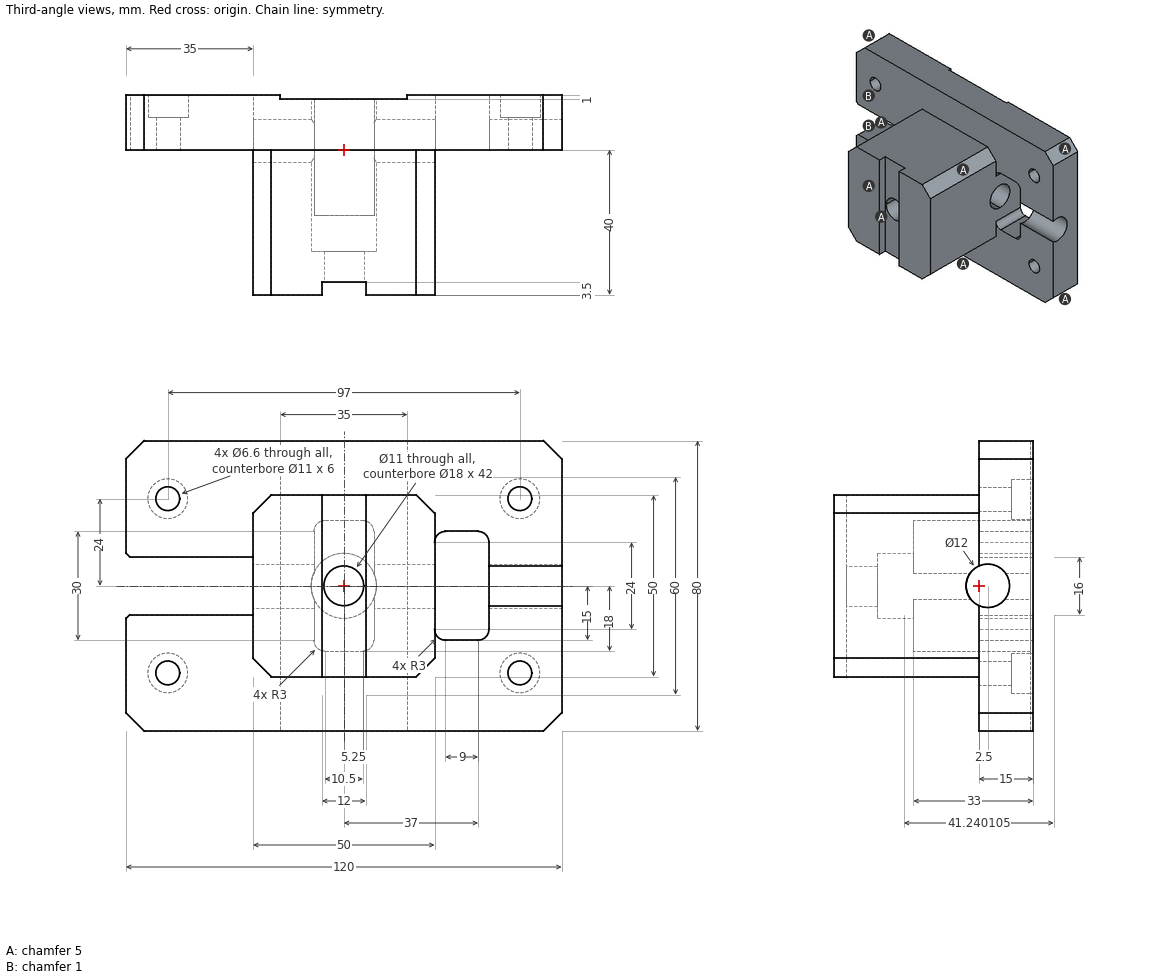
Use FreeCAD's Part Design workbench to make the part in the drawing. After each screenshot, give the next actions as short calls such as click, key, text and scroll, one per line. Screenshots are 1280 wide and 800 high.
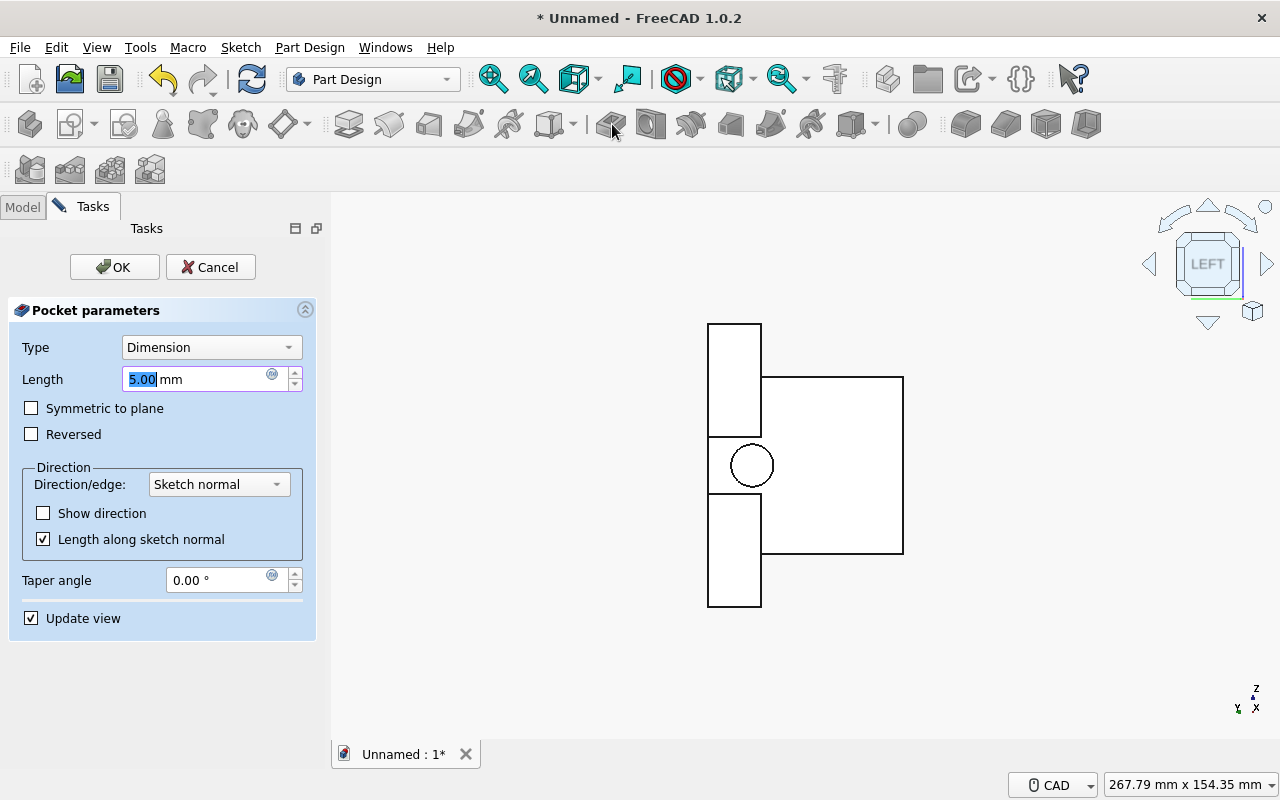
click(212, 348)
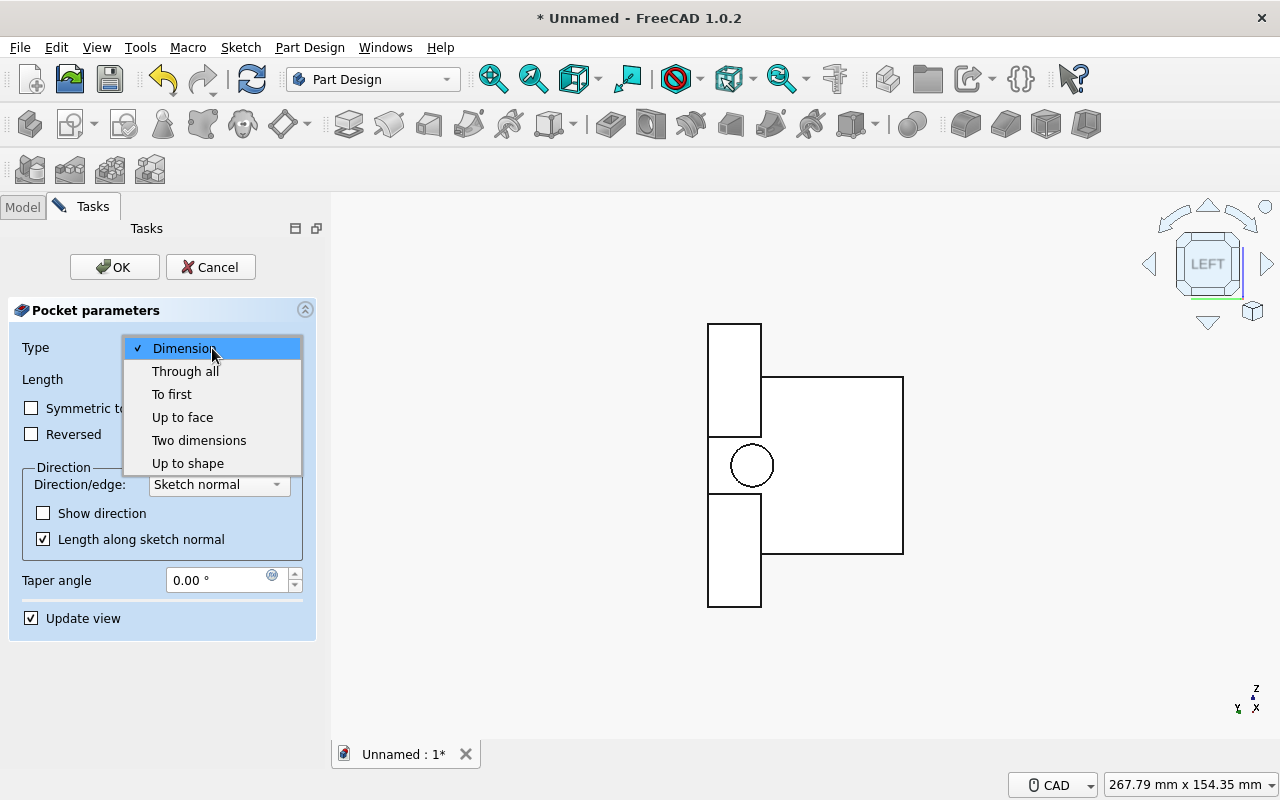
click(212, 372)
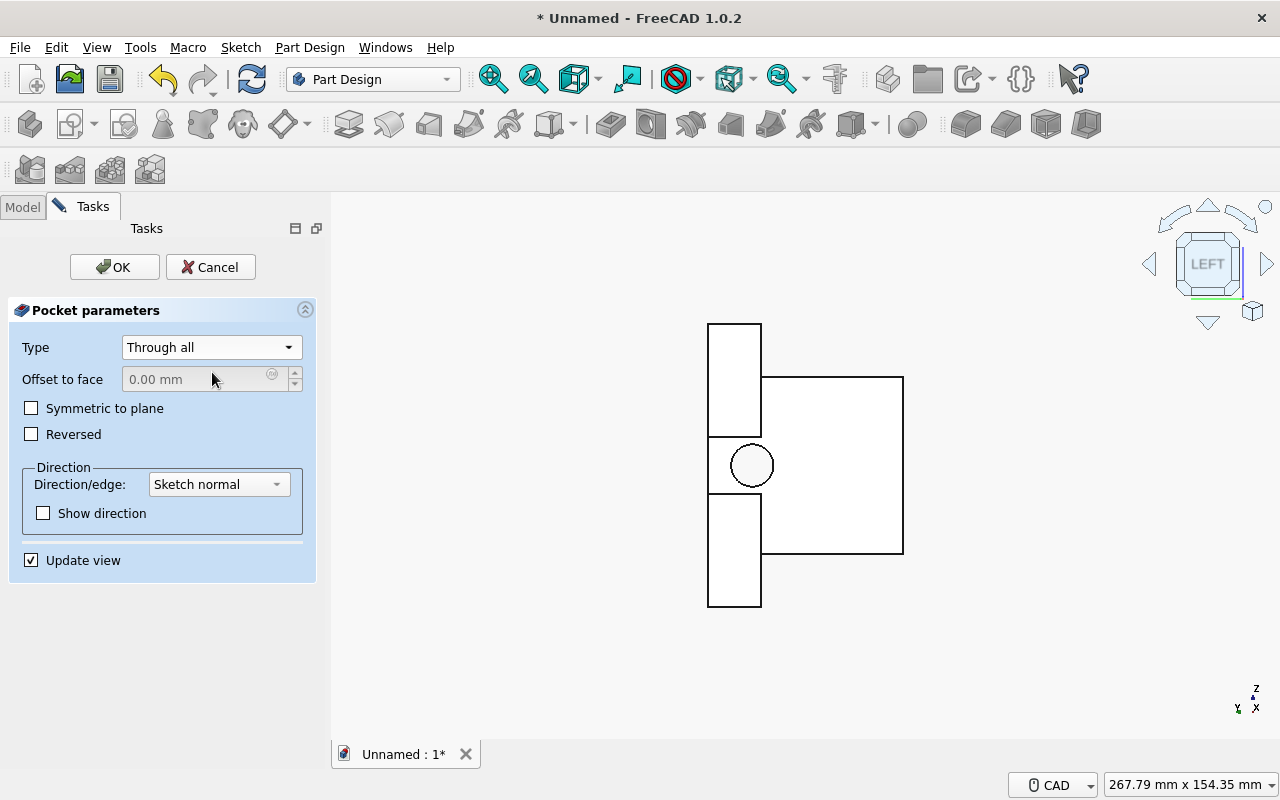
click(115, 267)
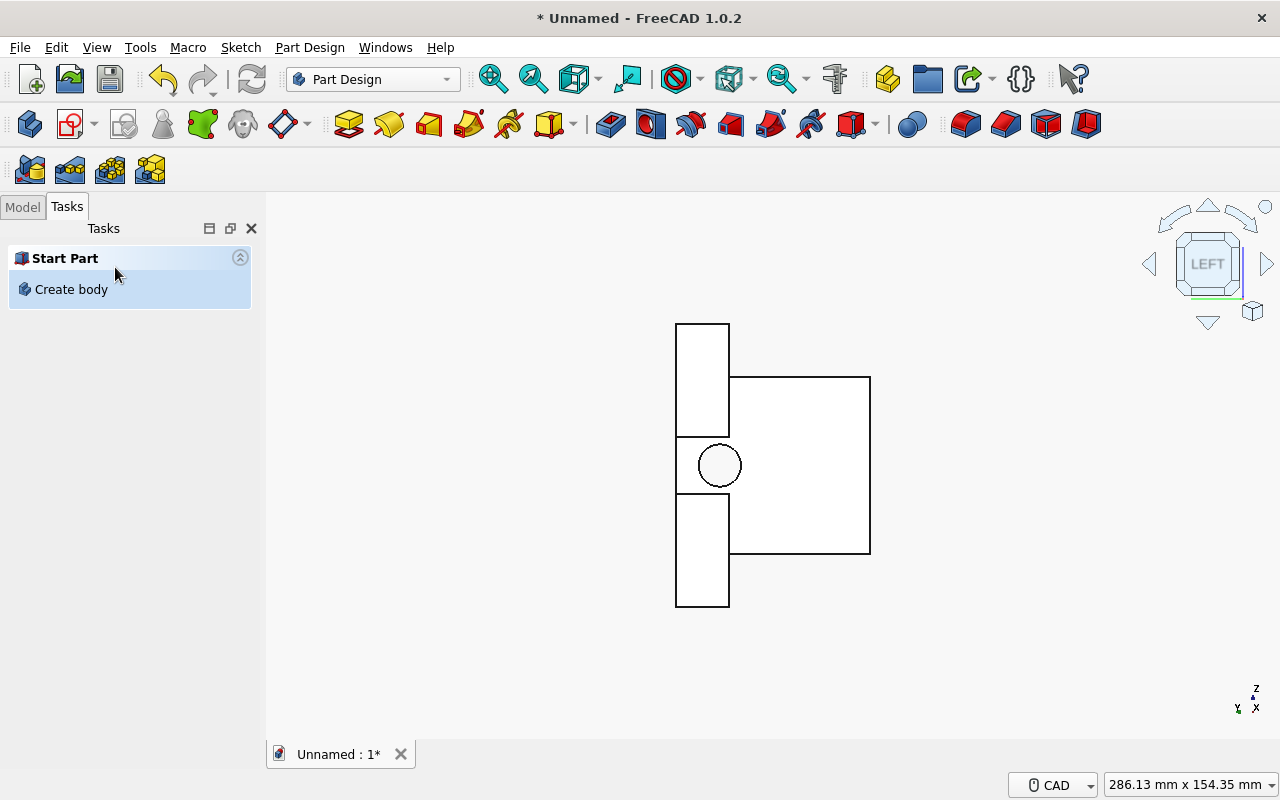
key(4)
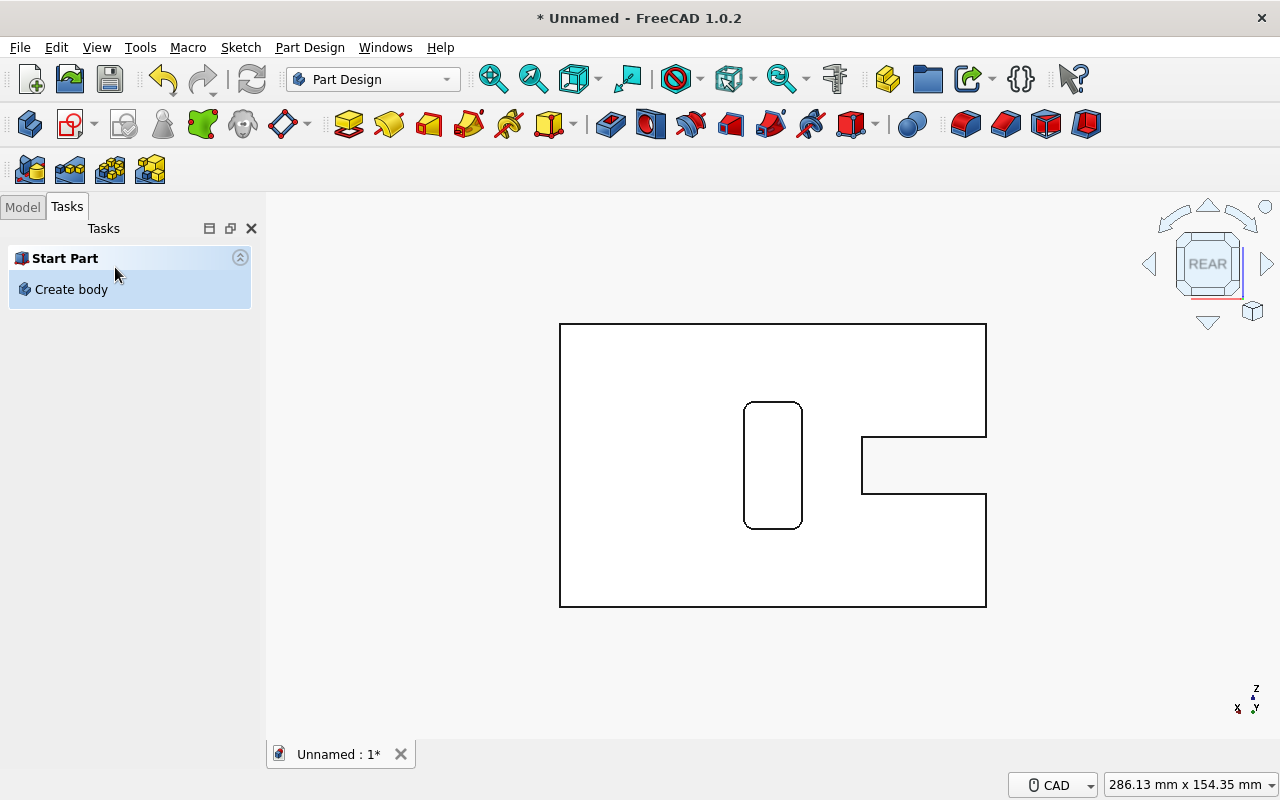
click(651, 424)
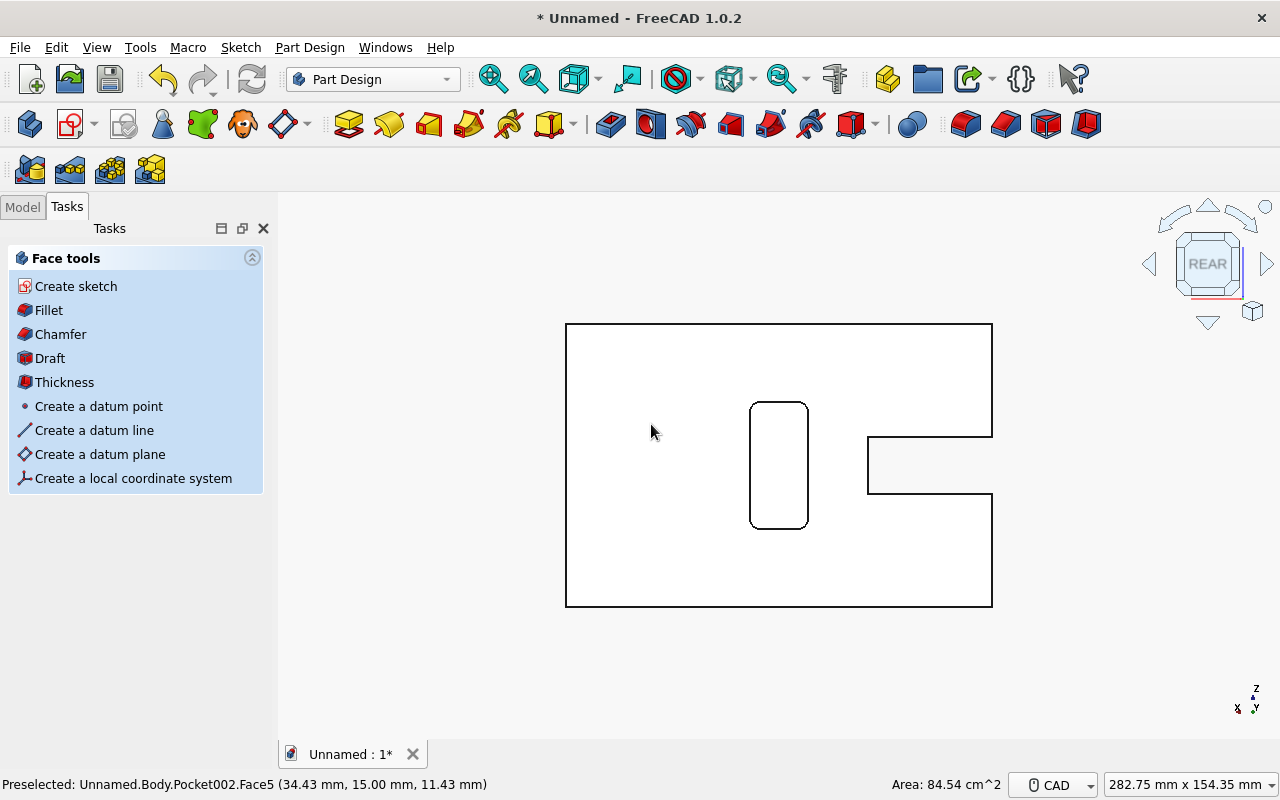
click(70, 124)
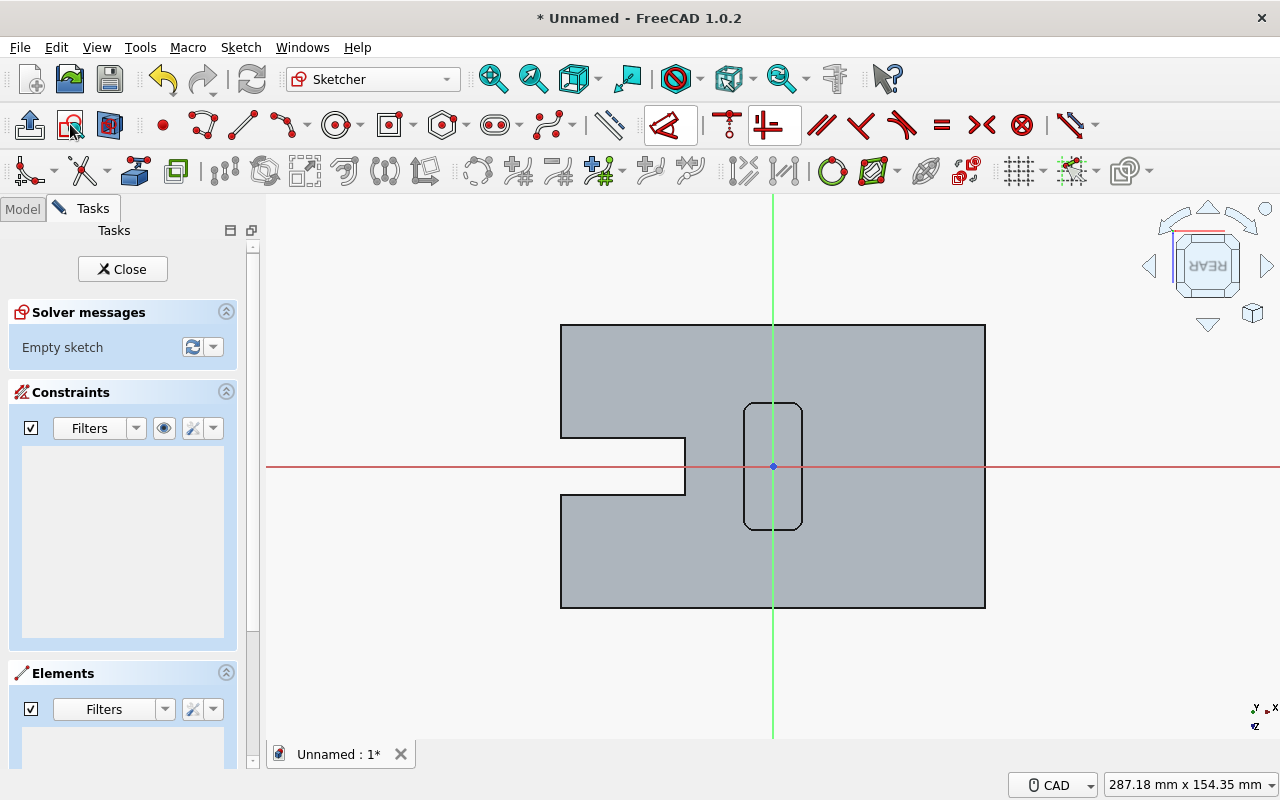
scroll(912, 466, up, 2)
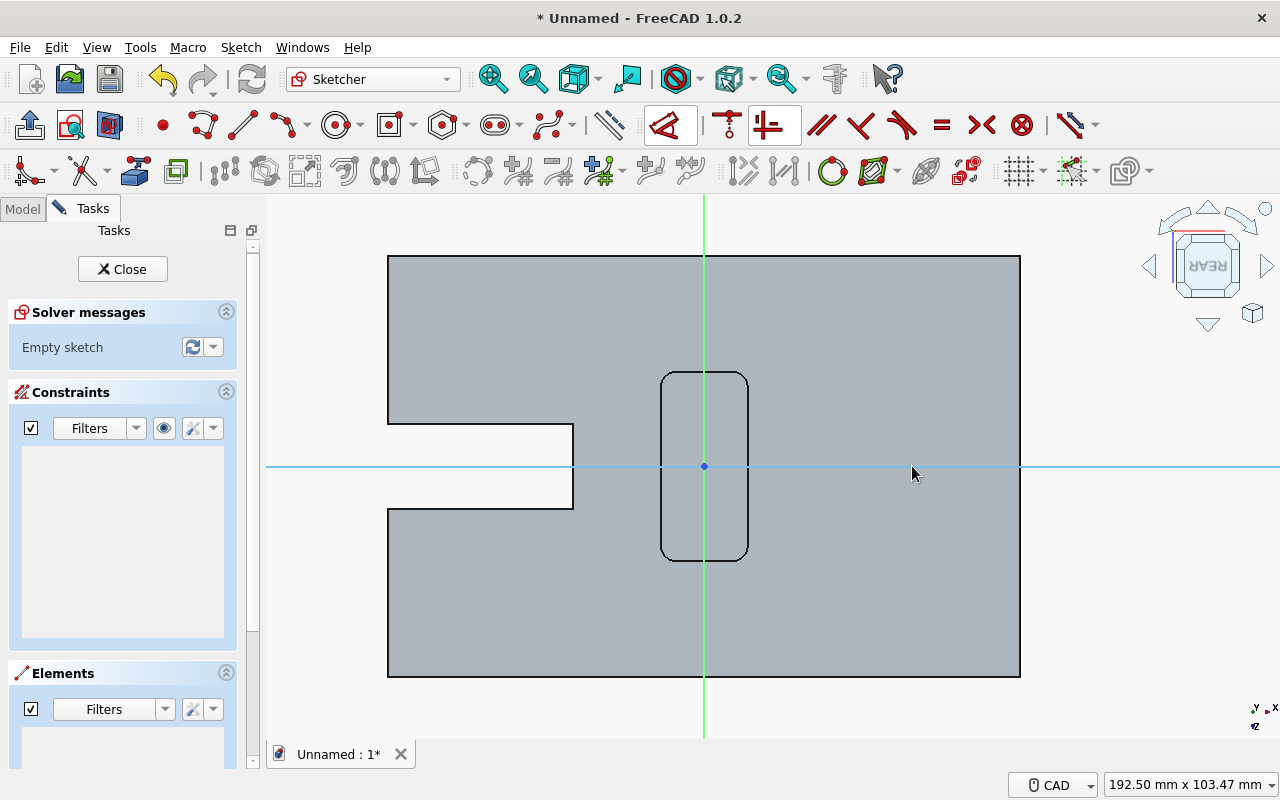
click(336, 126)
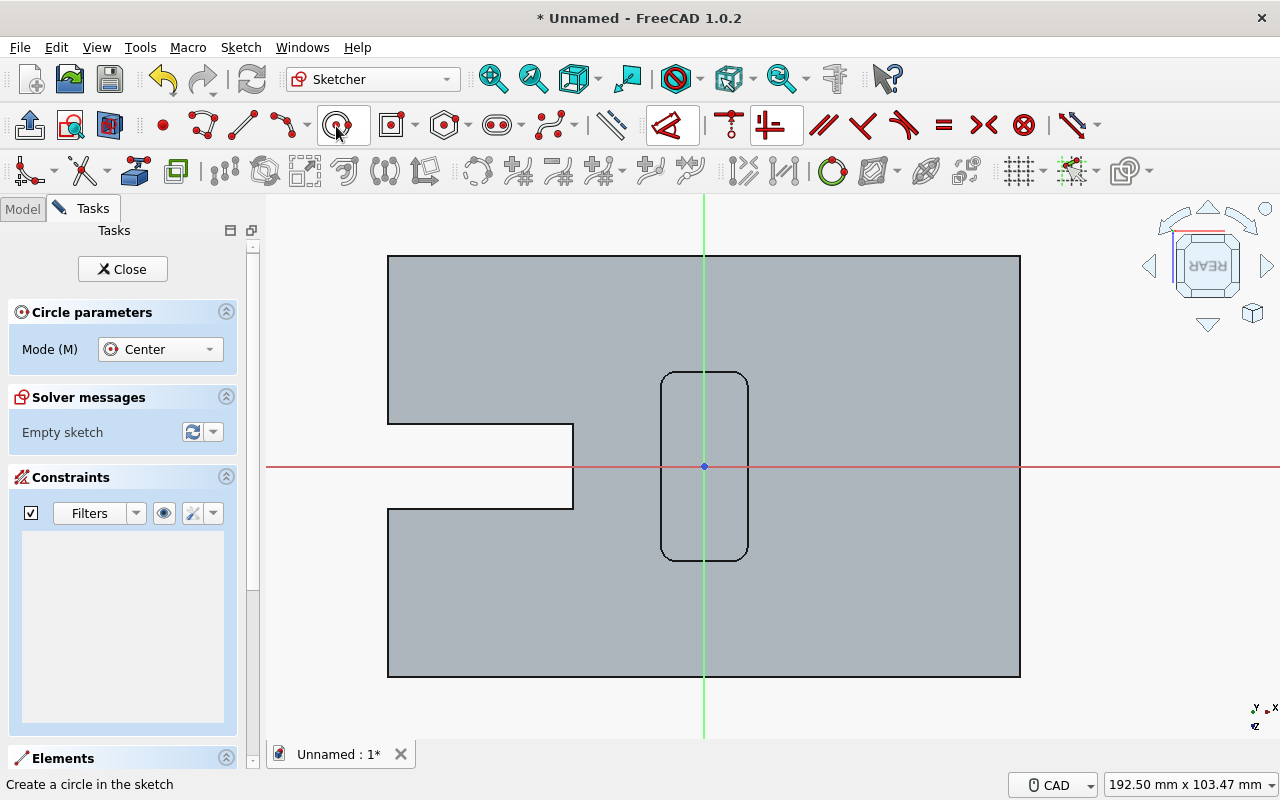
scroll(449, 593, up, 2)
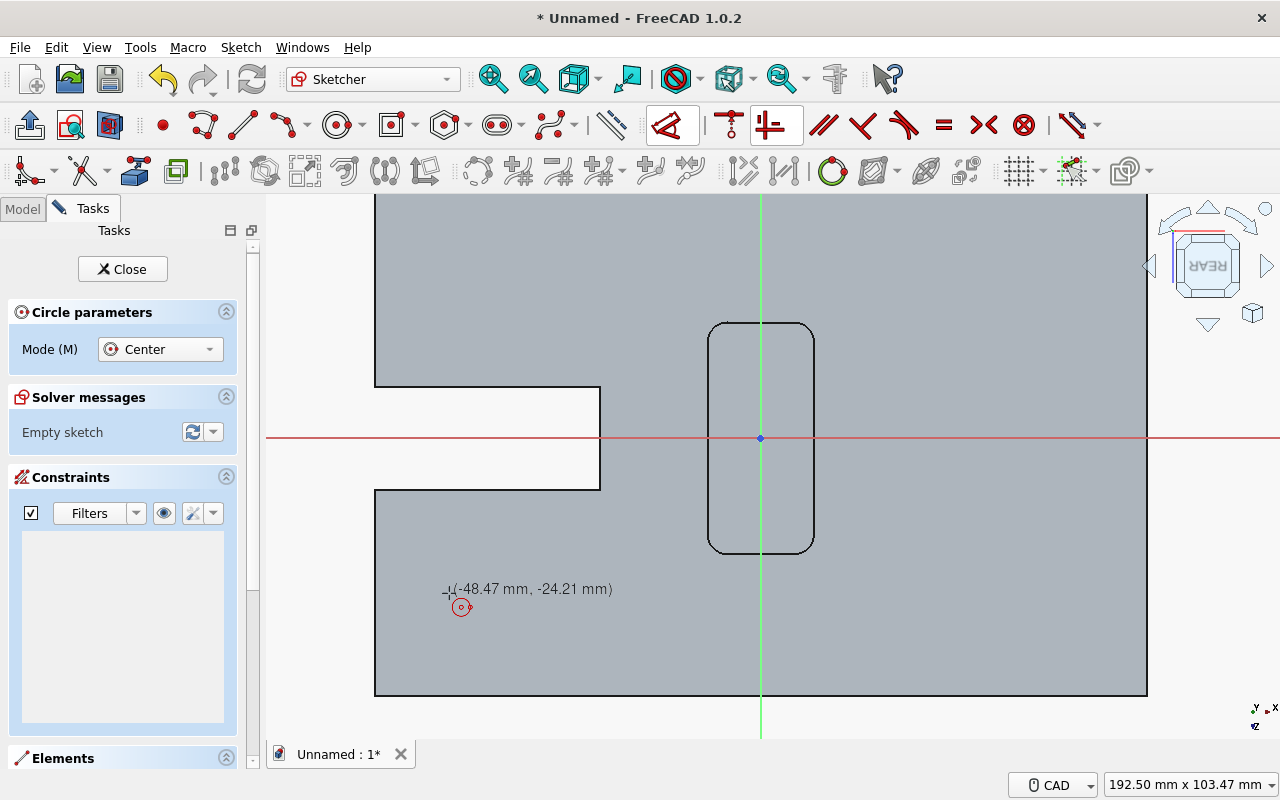
click(449, 593)
click(467, 574)